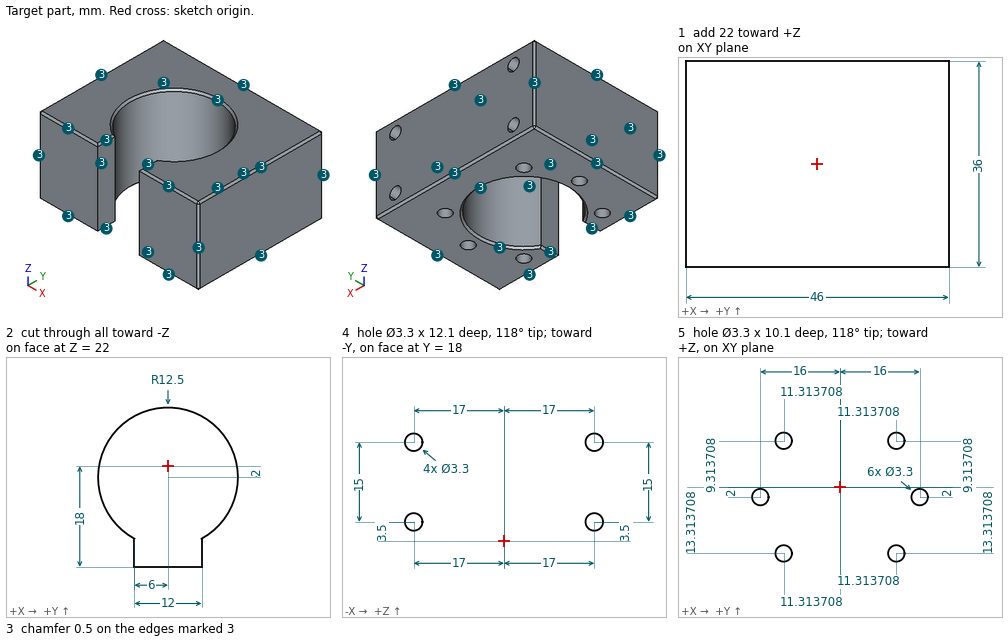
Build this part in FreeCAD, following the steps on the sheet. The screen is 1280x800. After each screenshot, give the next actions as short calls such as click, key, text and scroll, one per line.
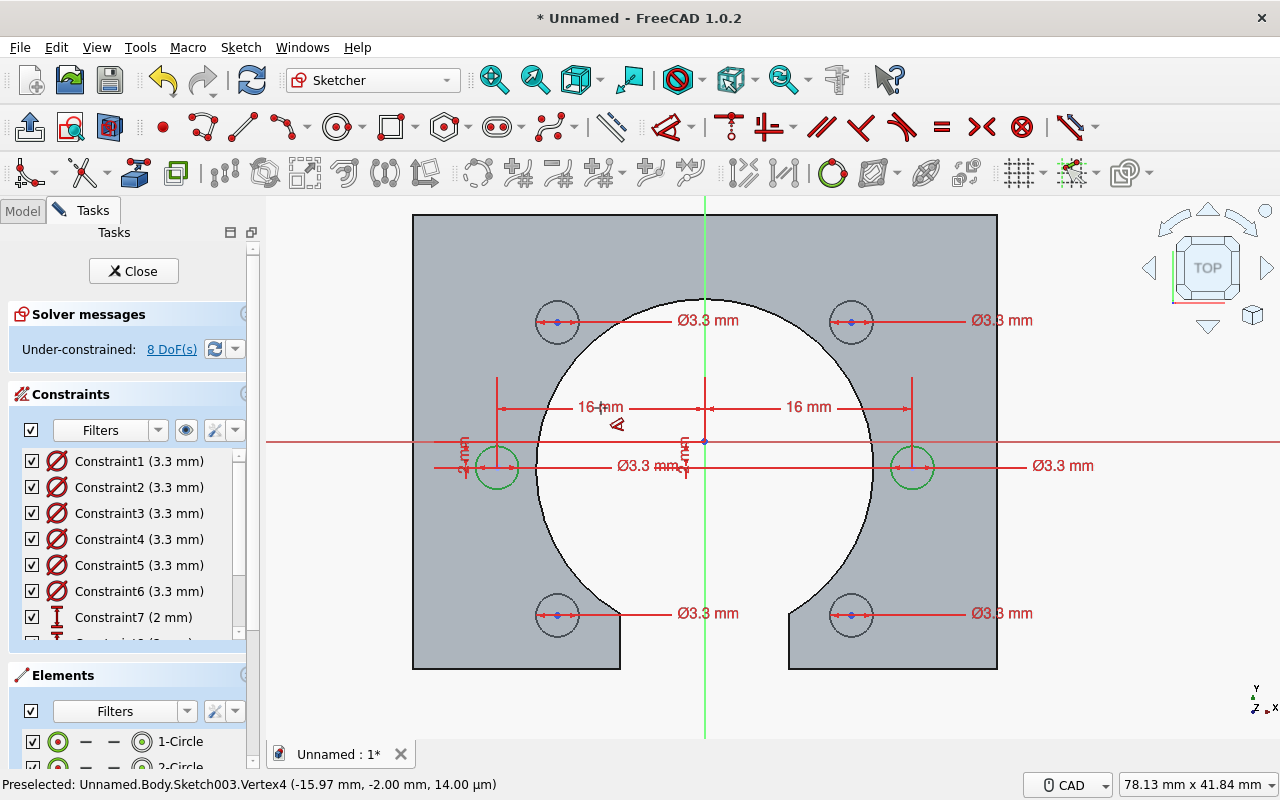
click(851, 322)
click(885, 382)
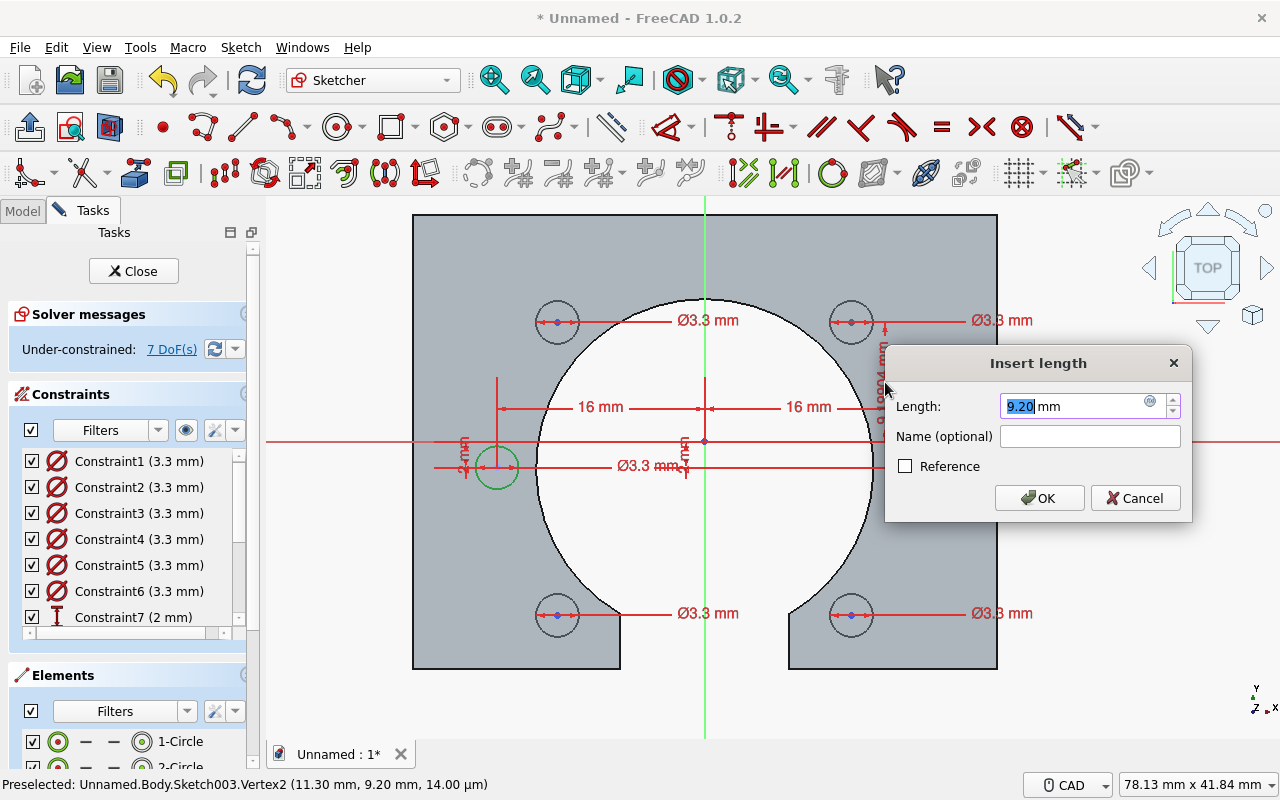
text(9.313708)
key(Return)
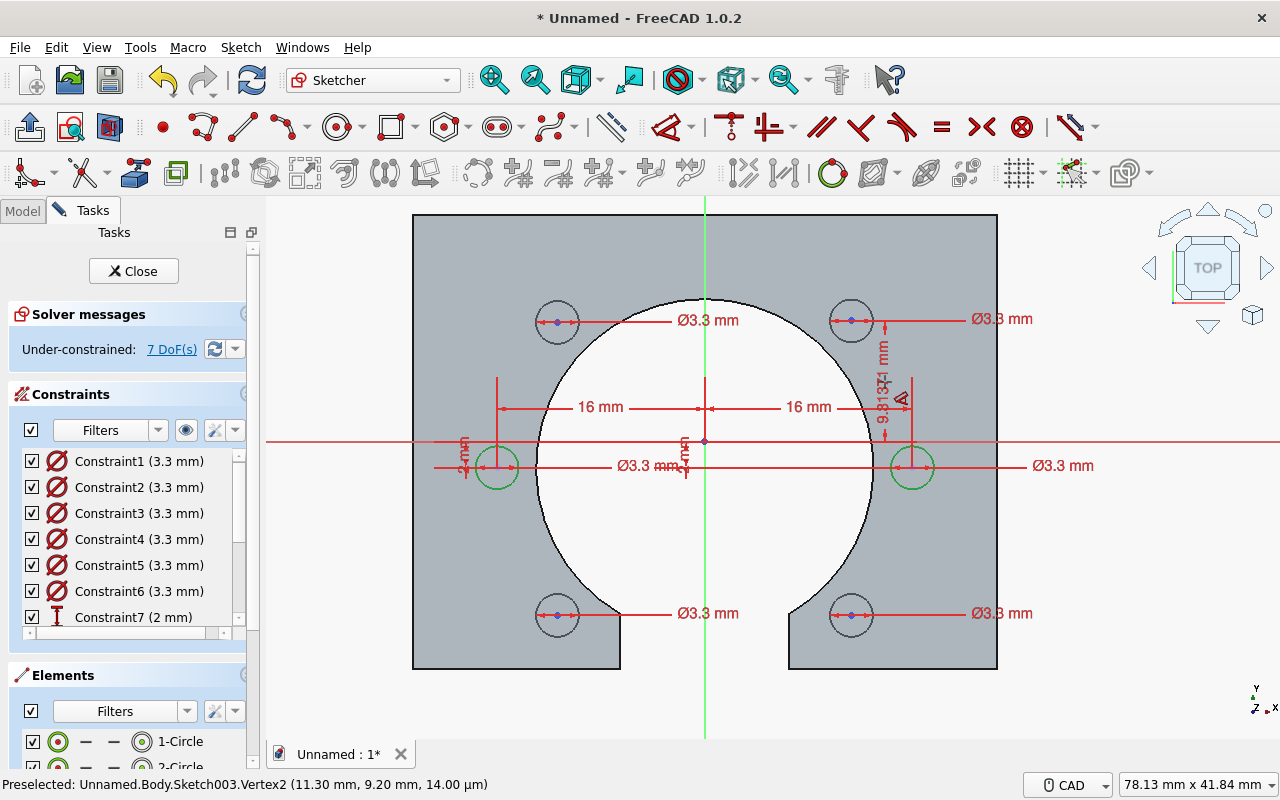
click(557, 322)
click(523, 382)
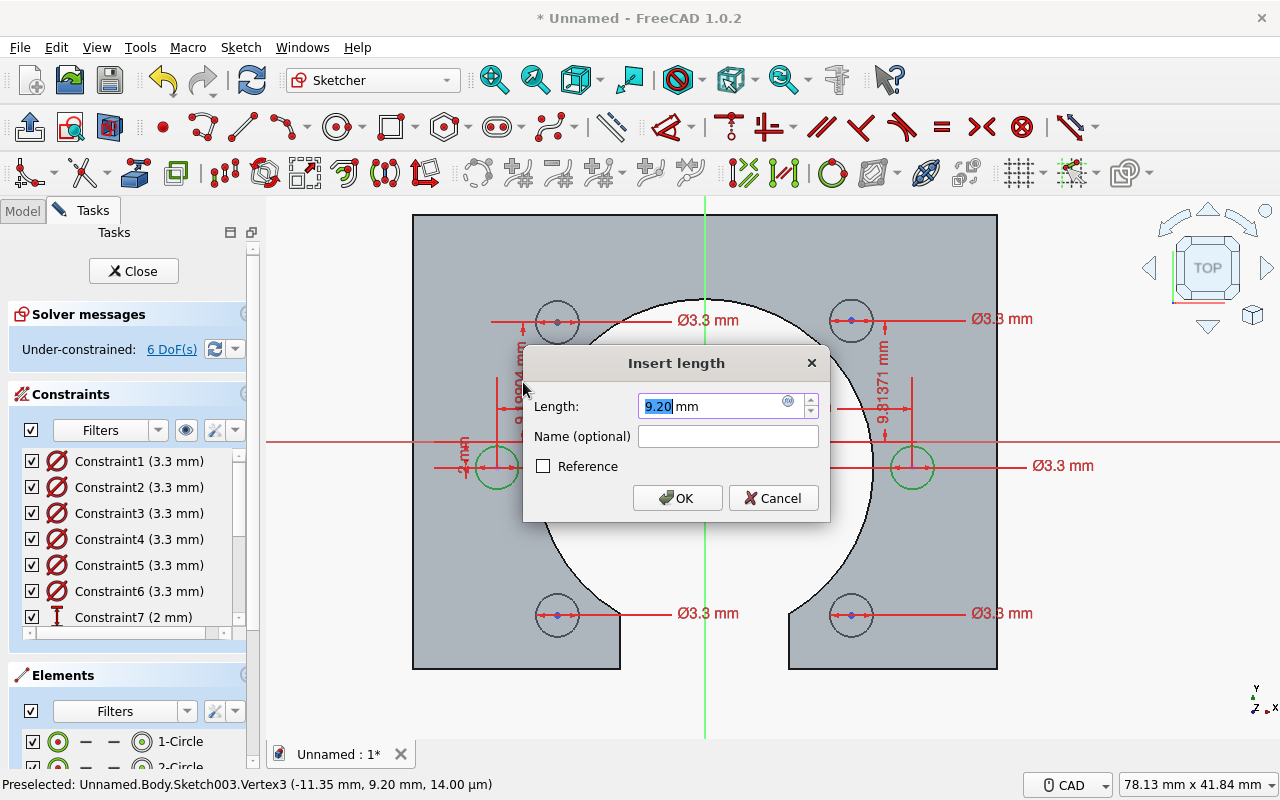
text(9.313708)
key(Return)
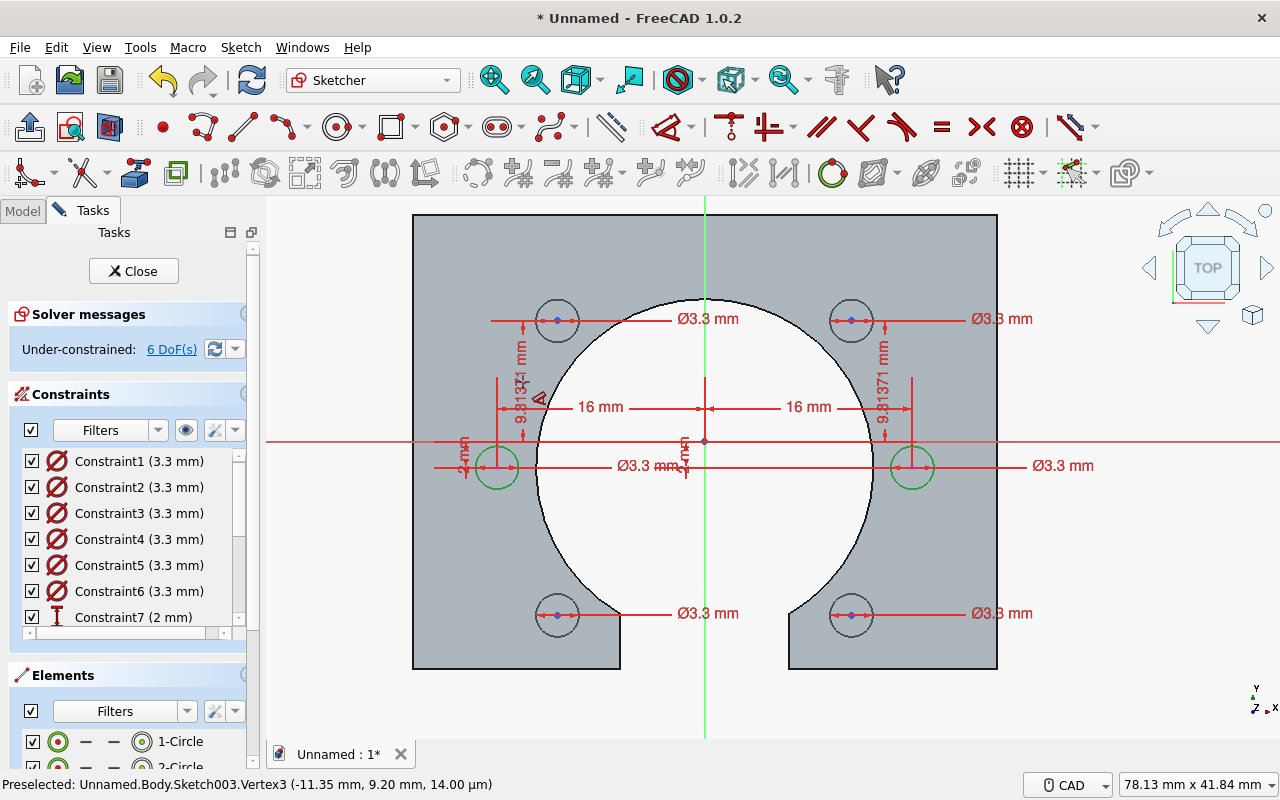
click(851, 321)
click(778, 287)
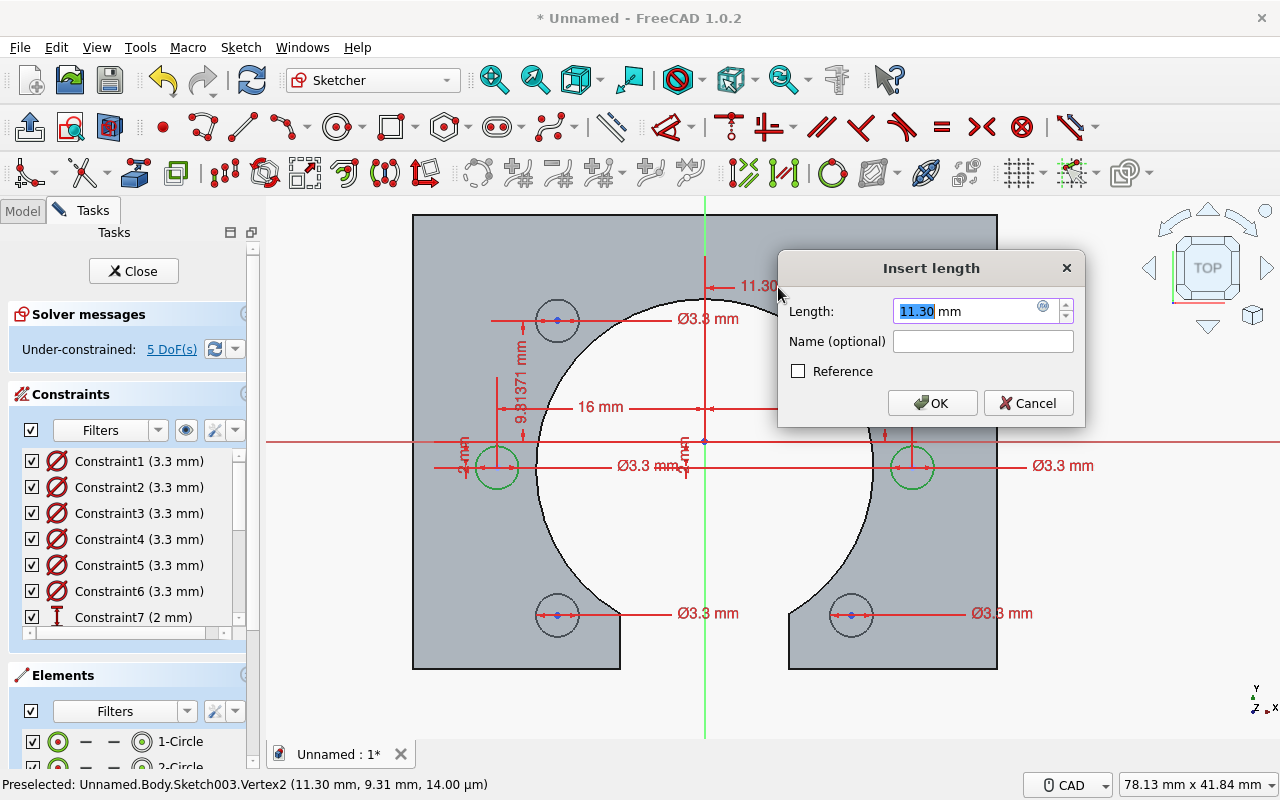
text(11.313708)
key(Return)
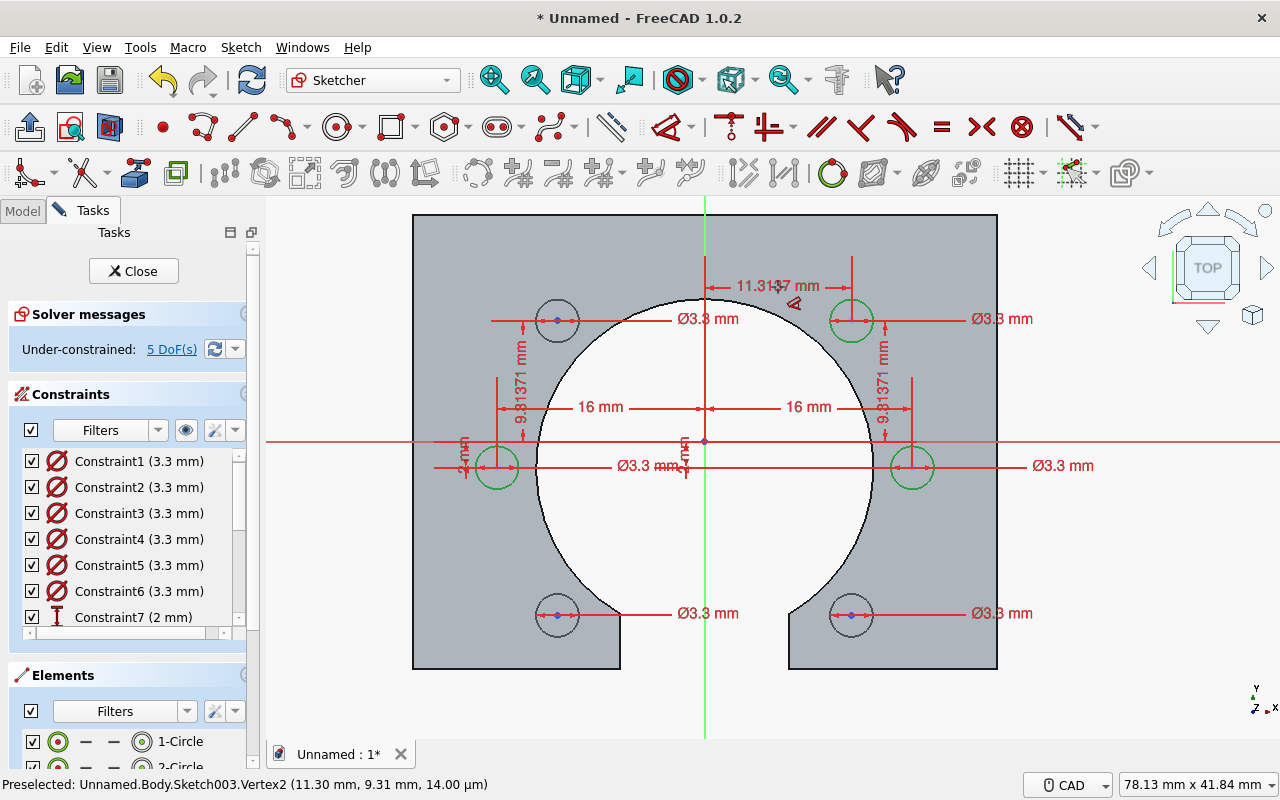
click(557, 321)
click(631, 287)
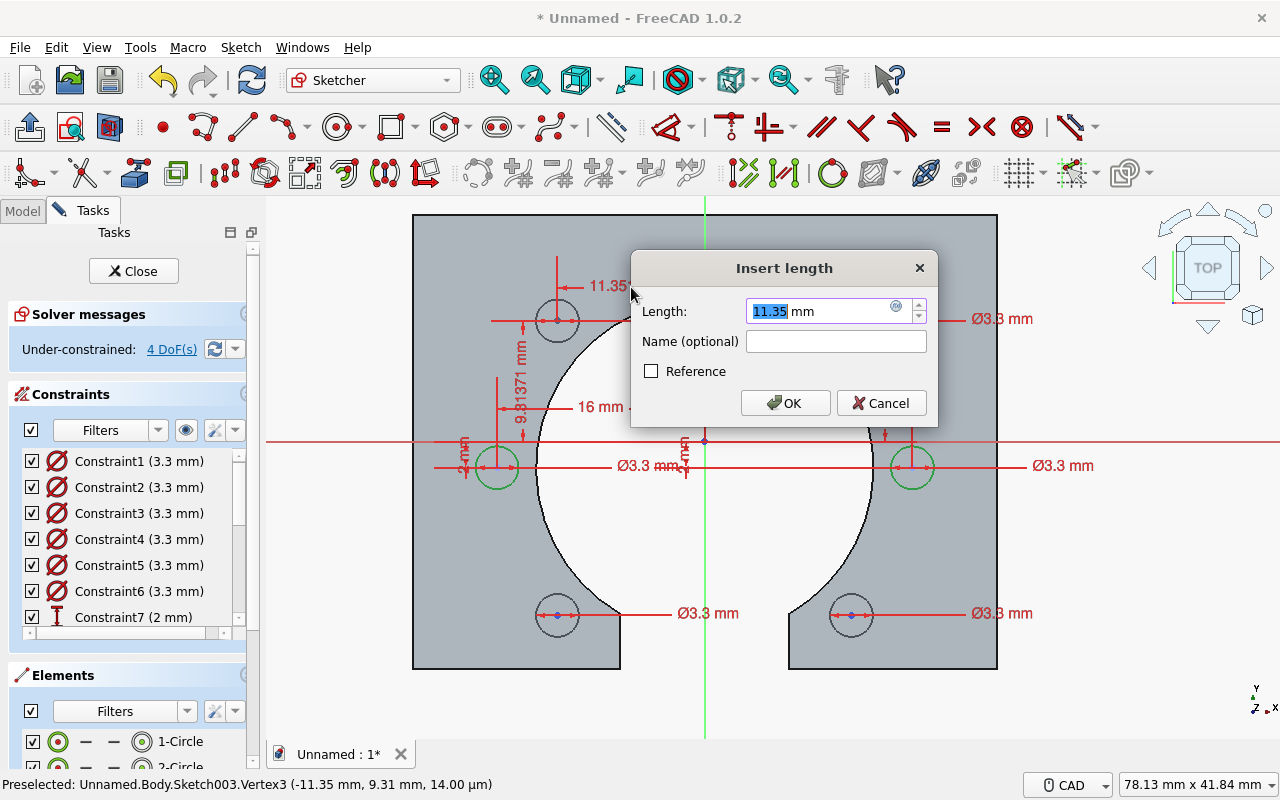
text(11.313708)
key(Return)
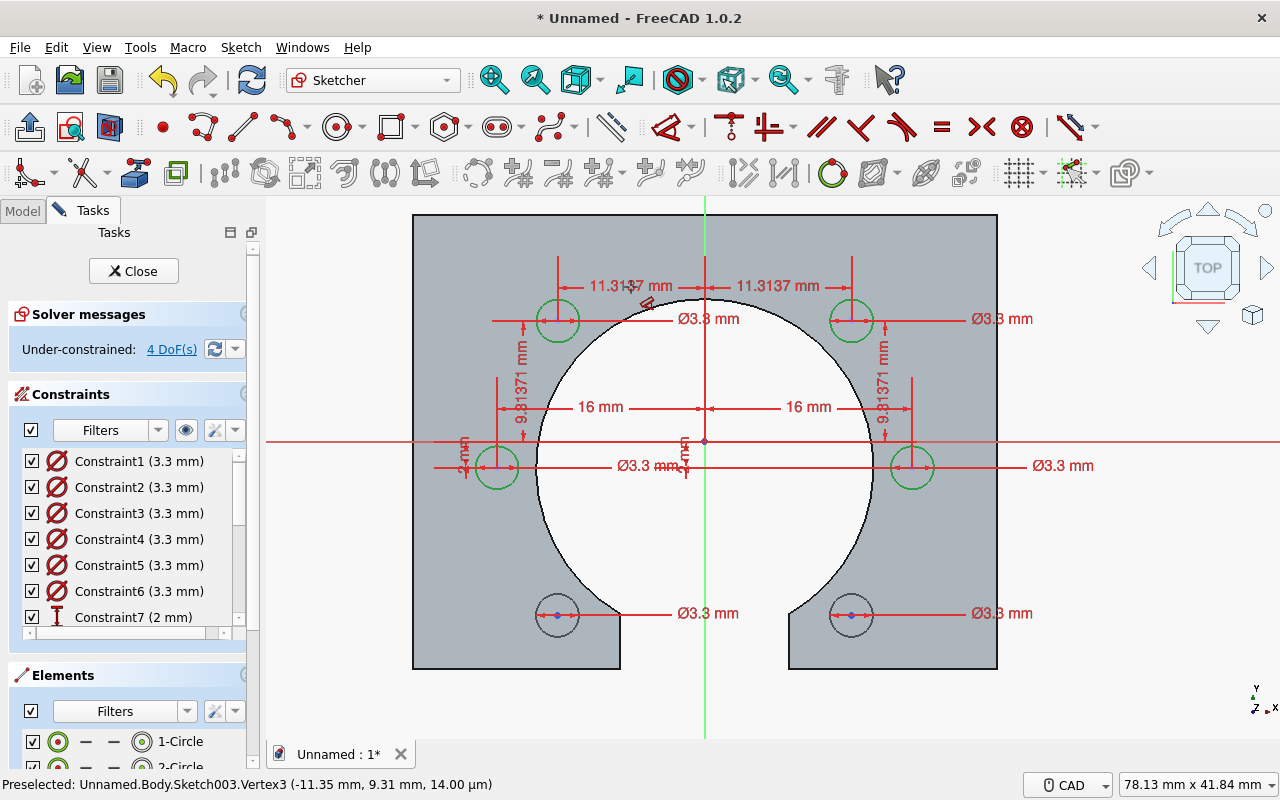
click(851, 615)
click(778, 649)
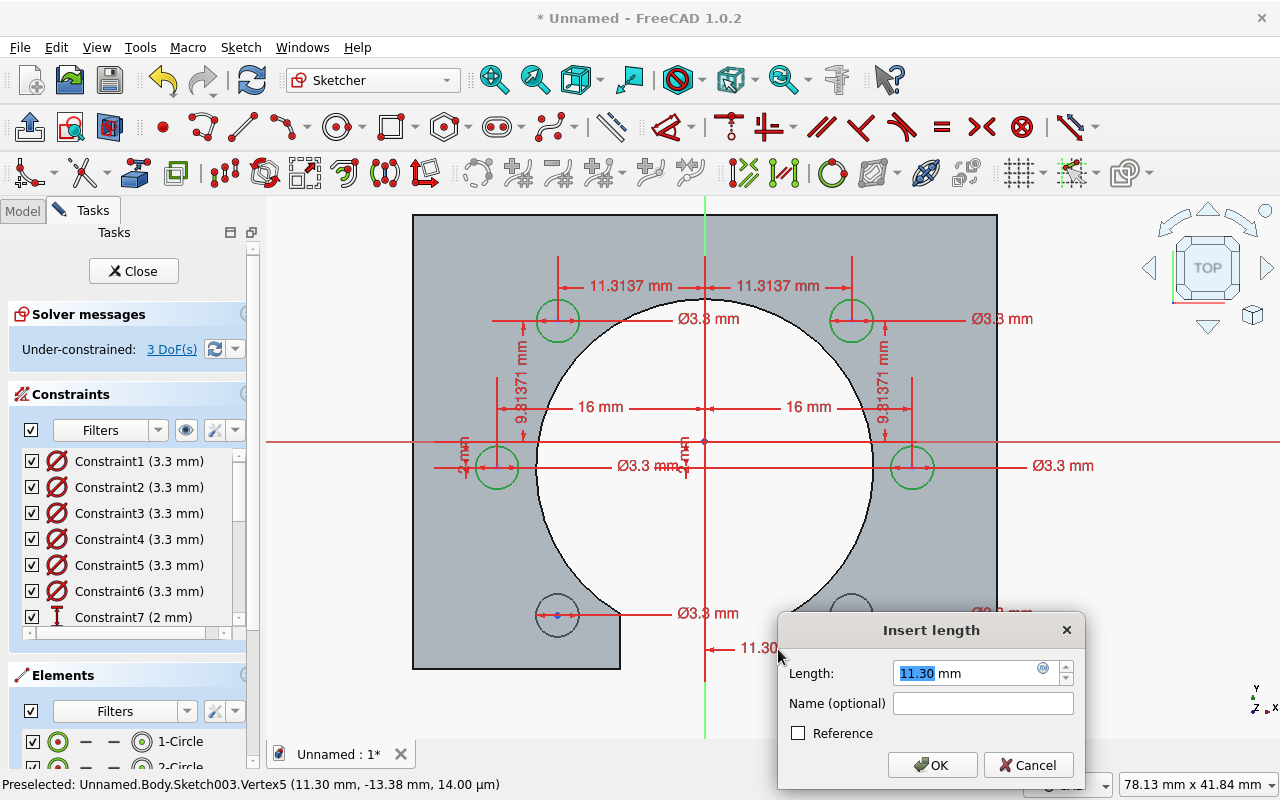
text(11.313708)
key(Return)